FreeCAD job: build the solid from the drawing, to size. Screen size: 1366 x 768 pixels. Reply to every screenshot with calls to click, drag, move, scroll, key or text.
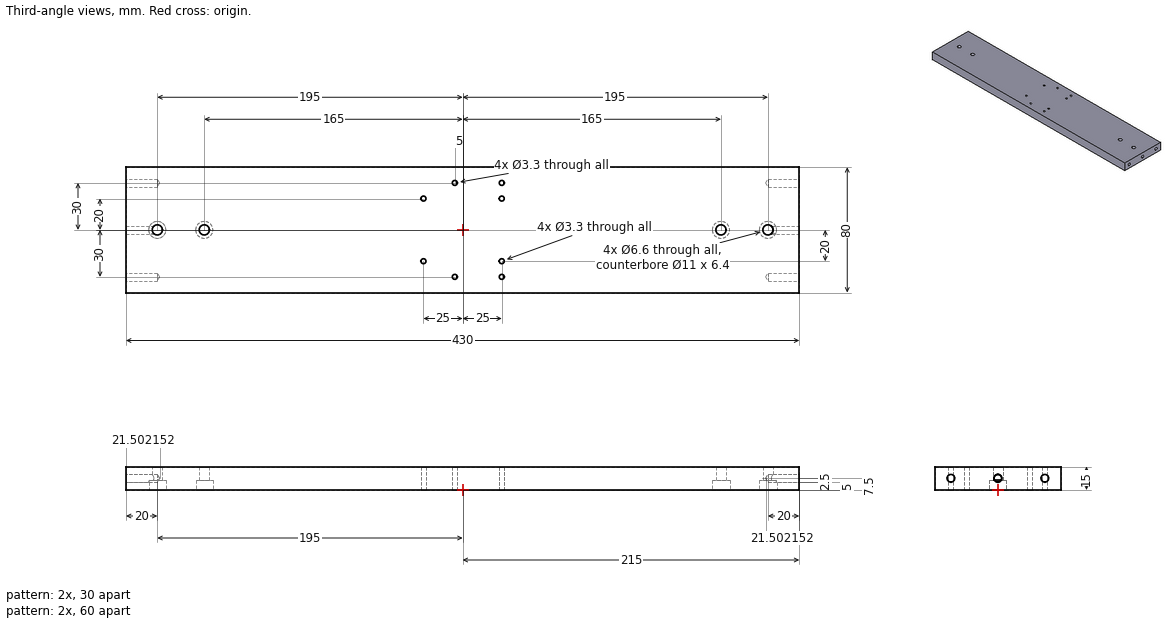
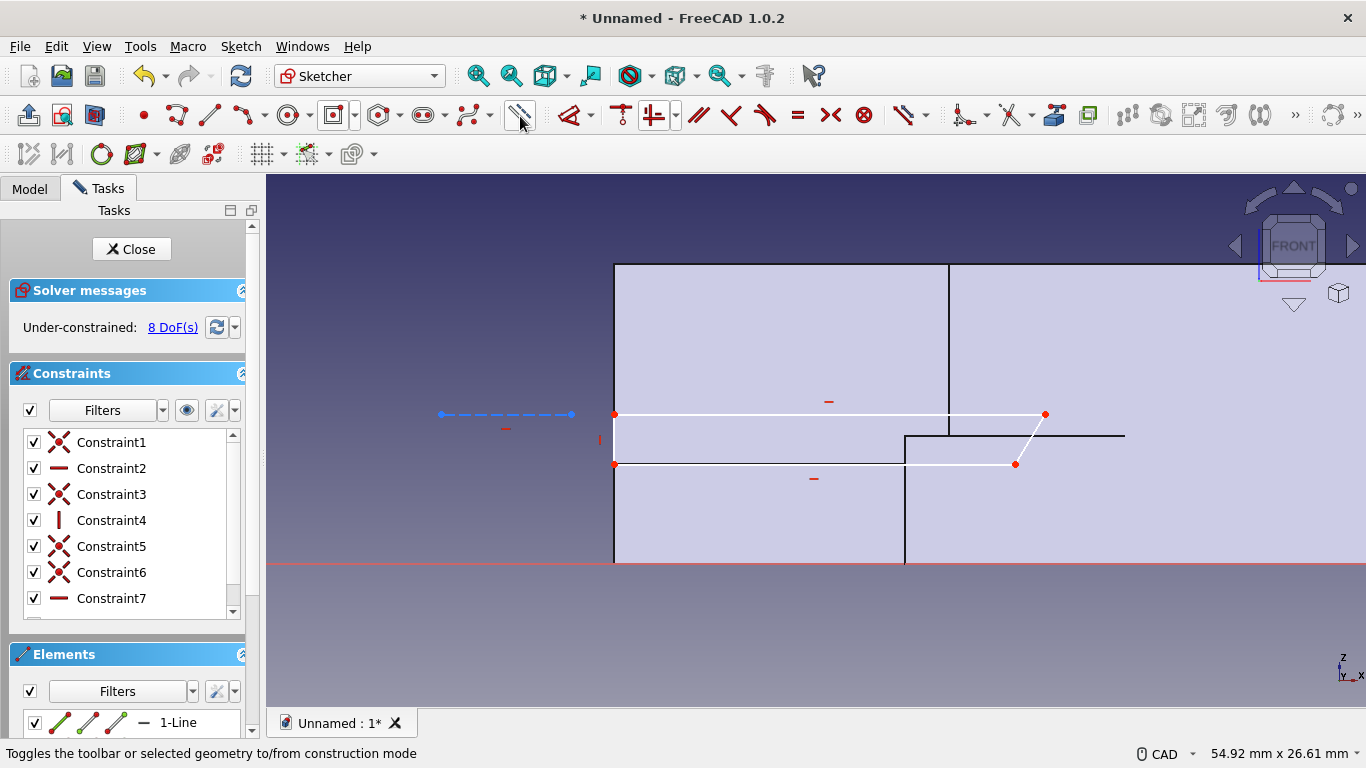
click(568, 116)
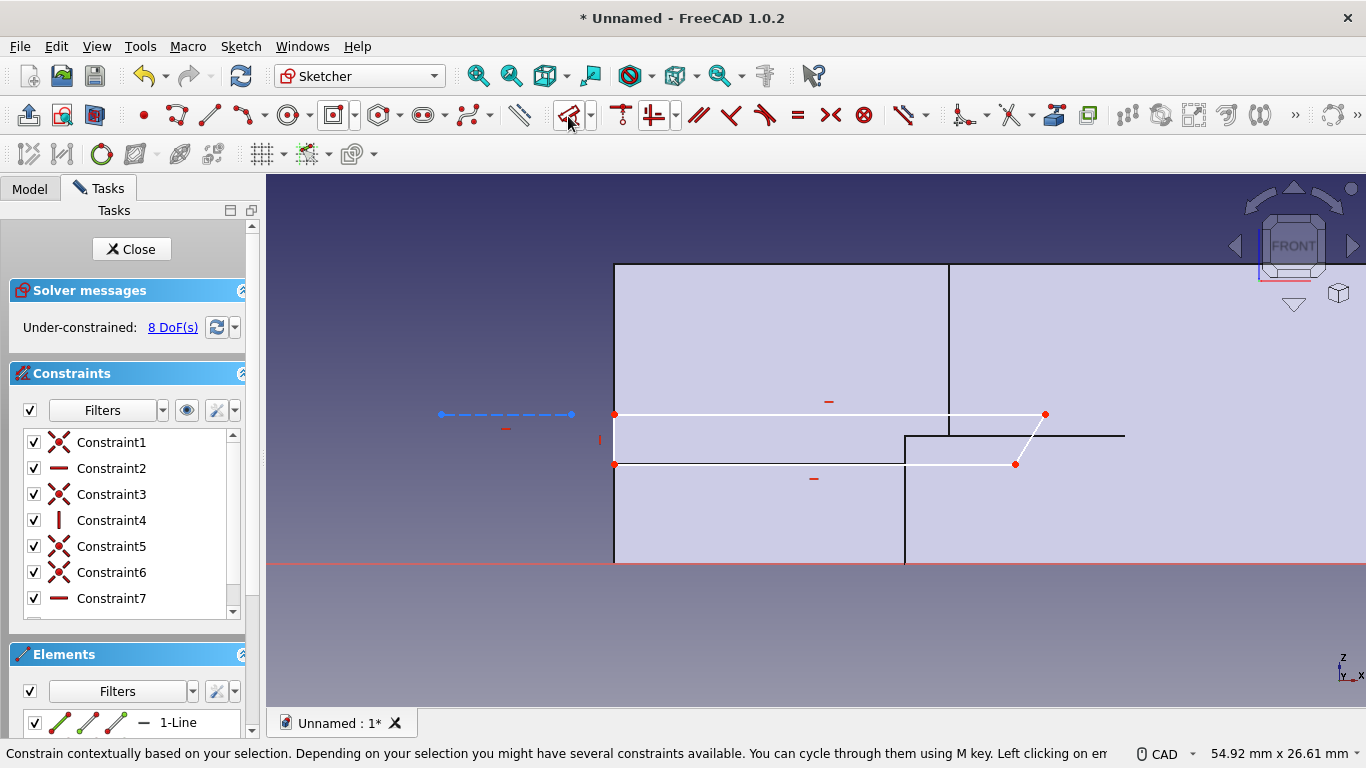
click(895, 465)
click(815, 499)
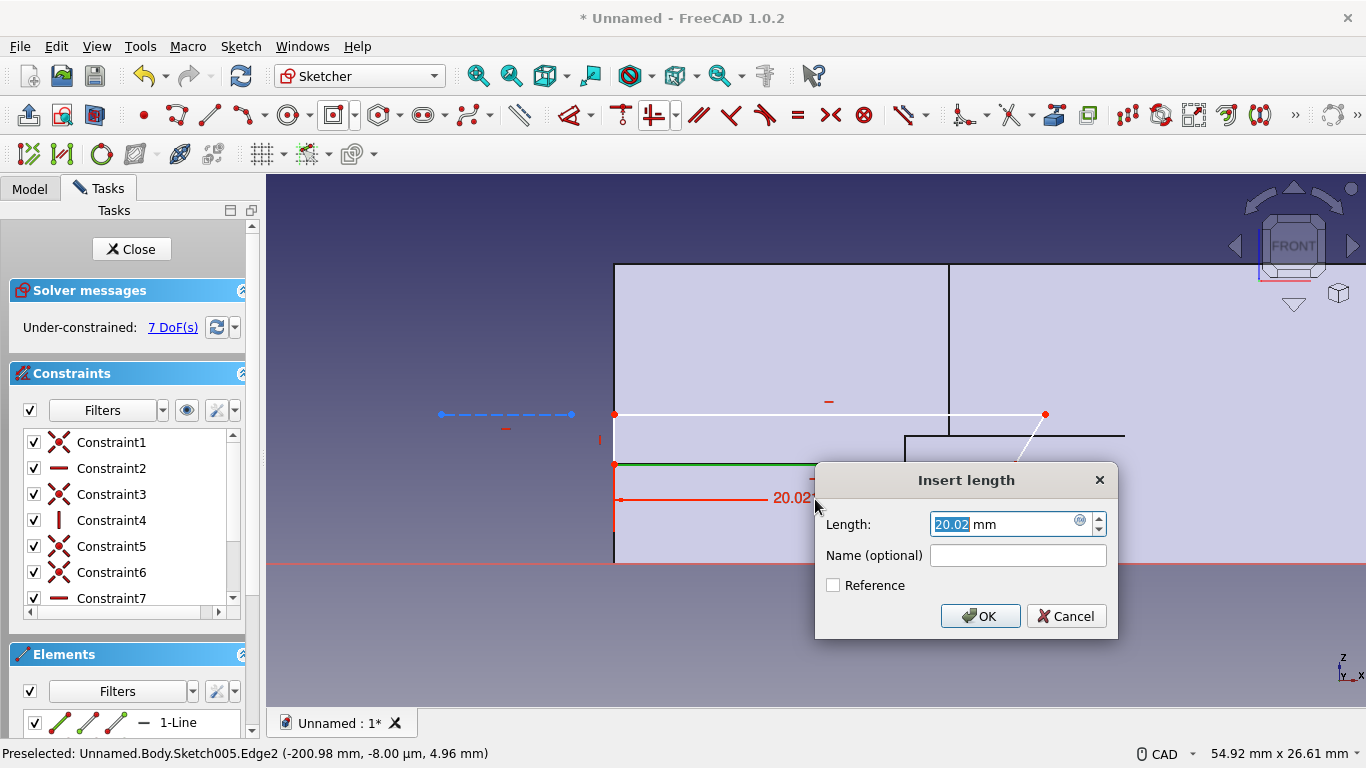
text(20)
key(Return)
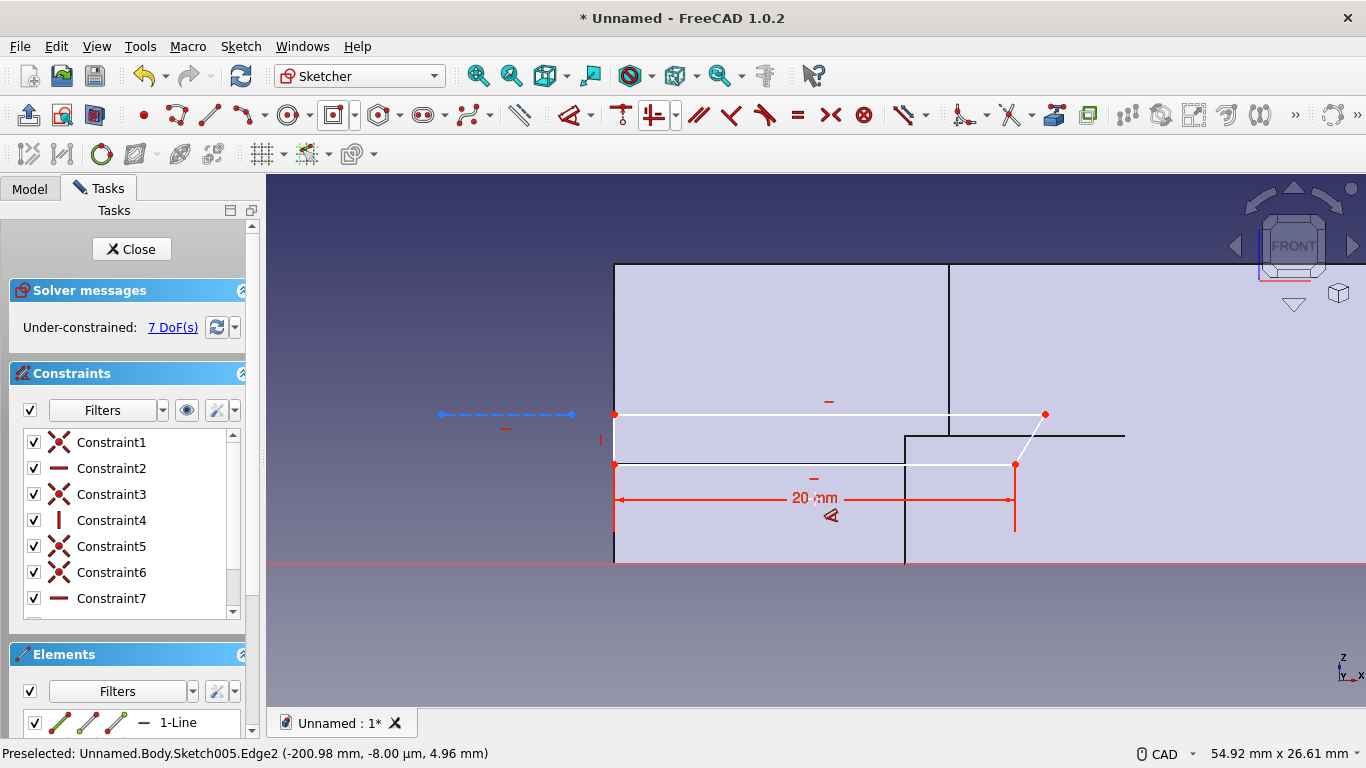
click(1015, 465)
click(981, 515)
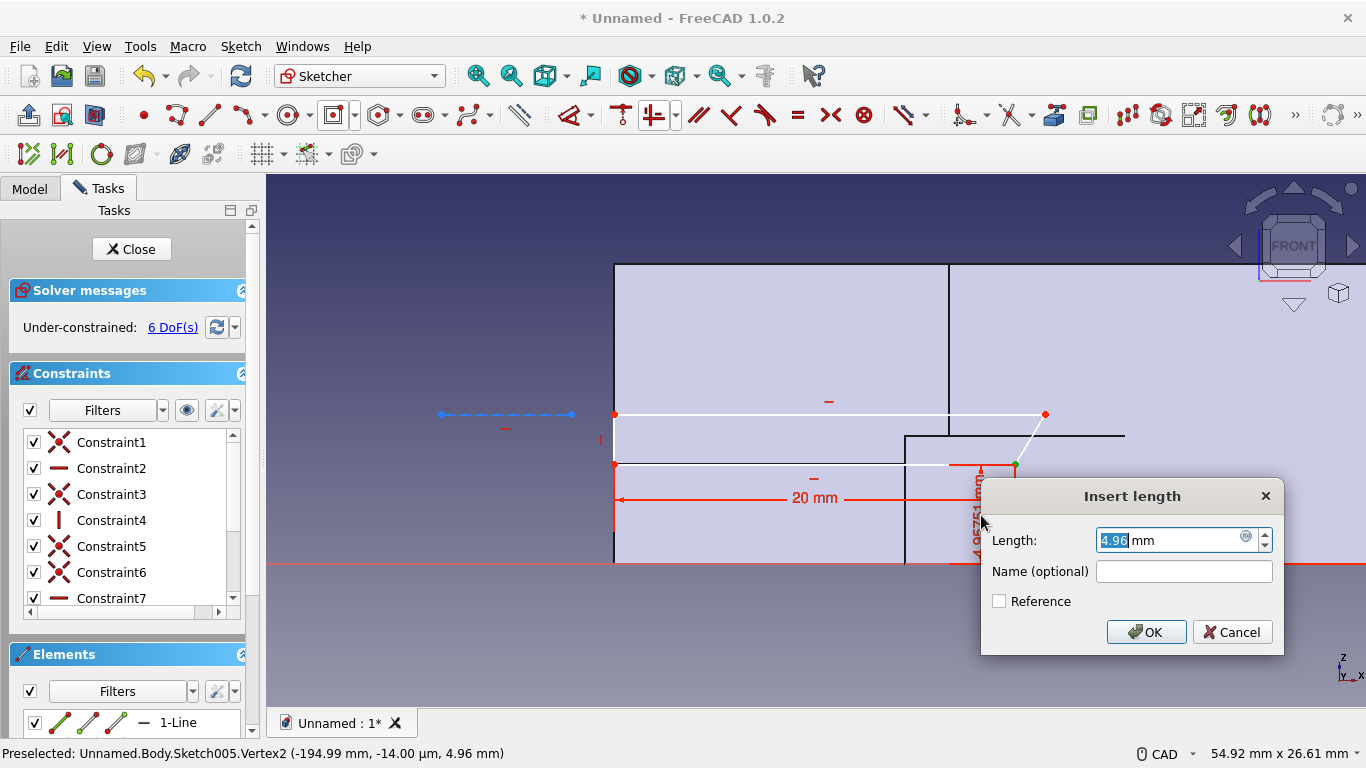
text(5)
key(Return)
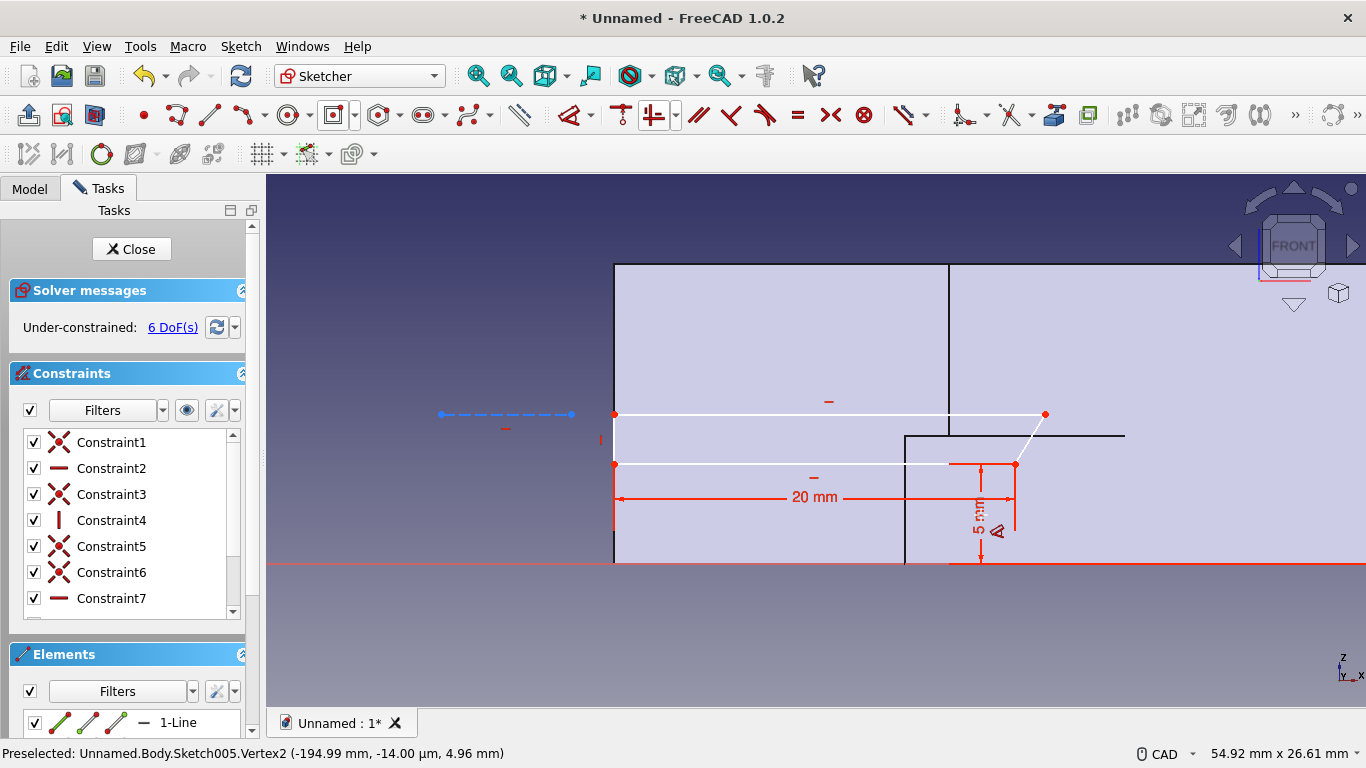
click(614, 449)
click(580, 440)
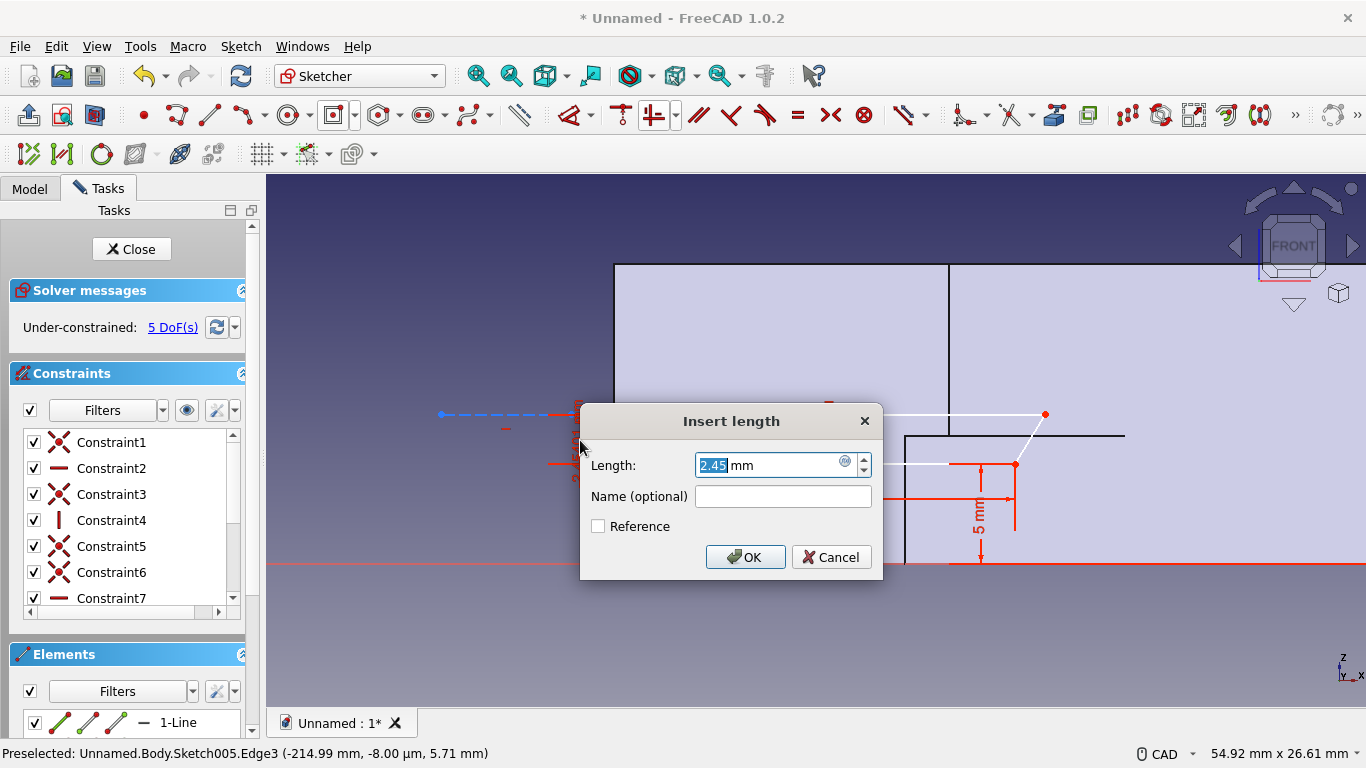
text(2.5)
key(Return)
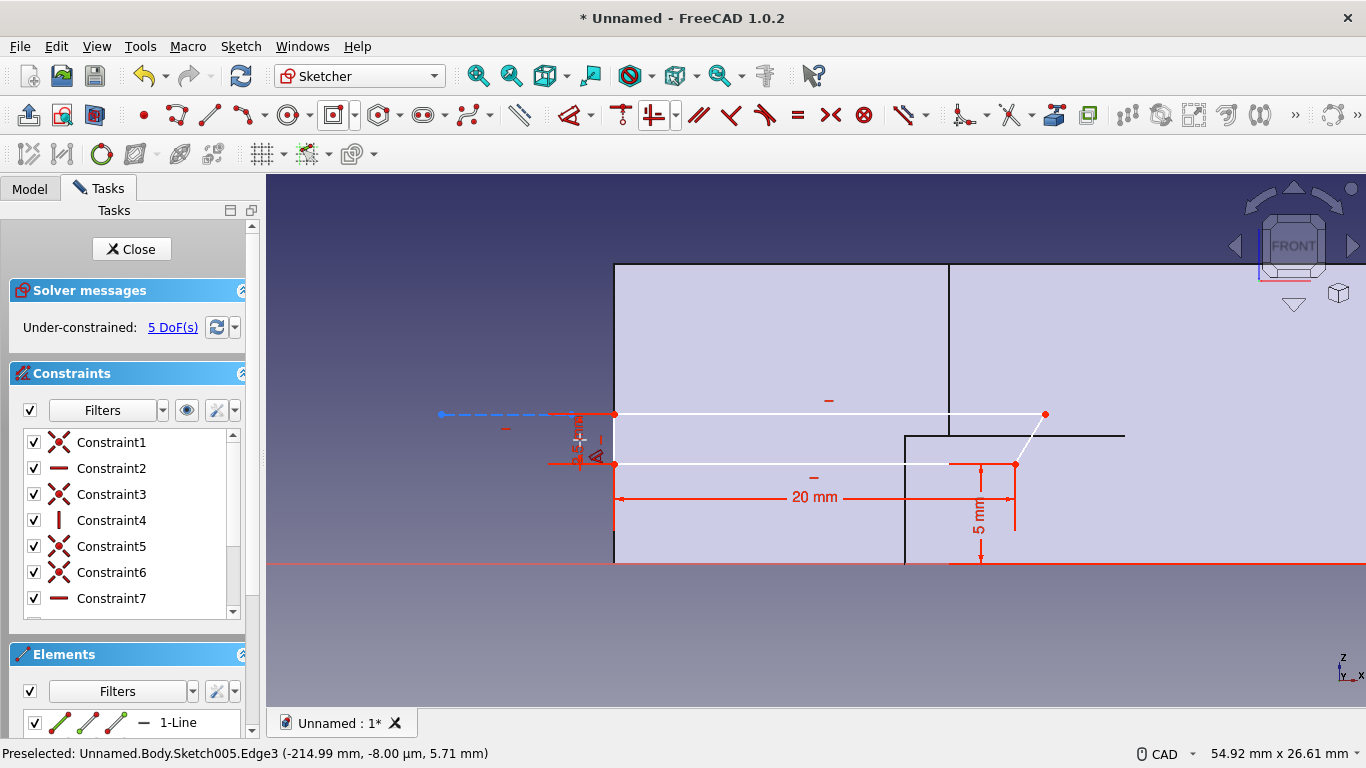
click(1015, 464)
click(1108, 598)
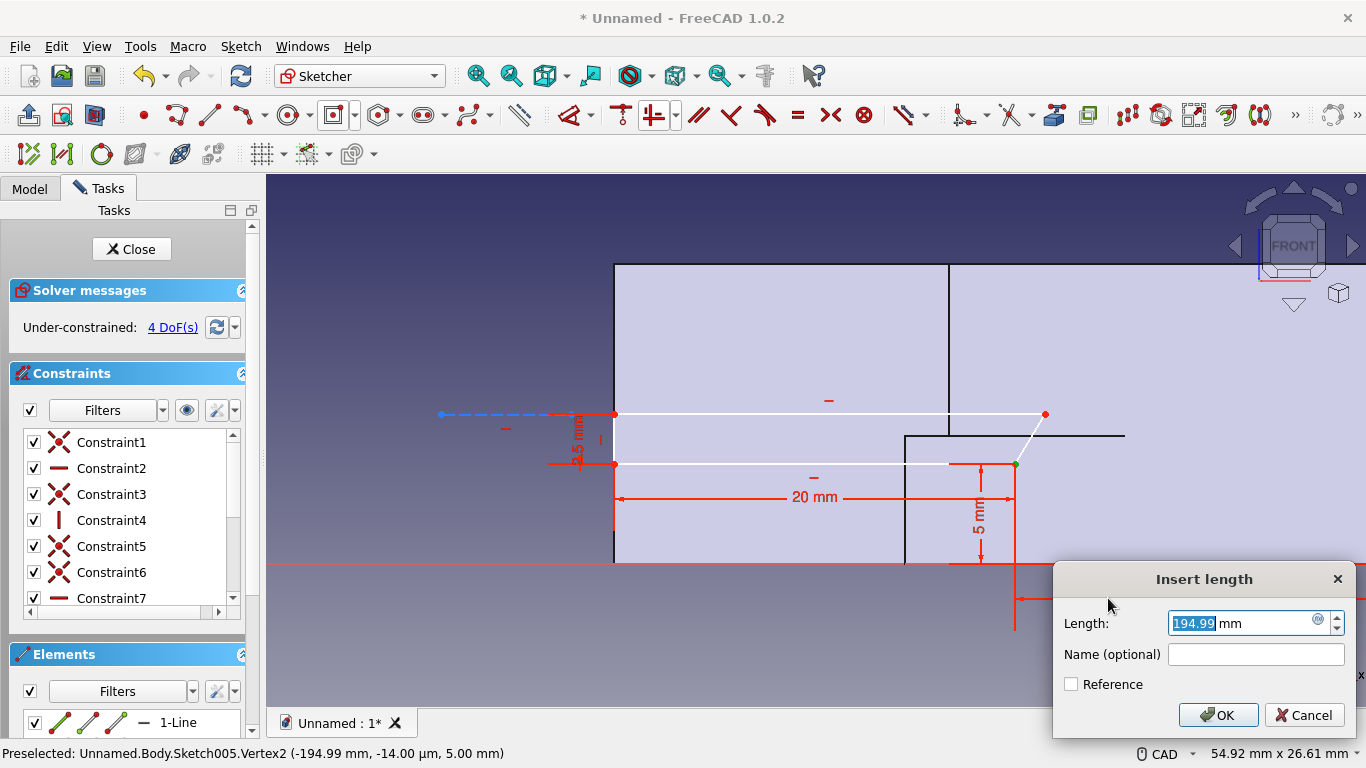
text(195)
key(Return)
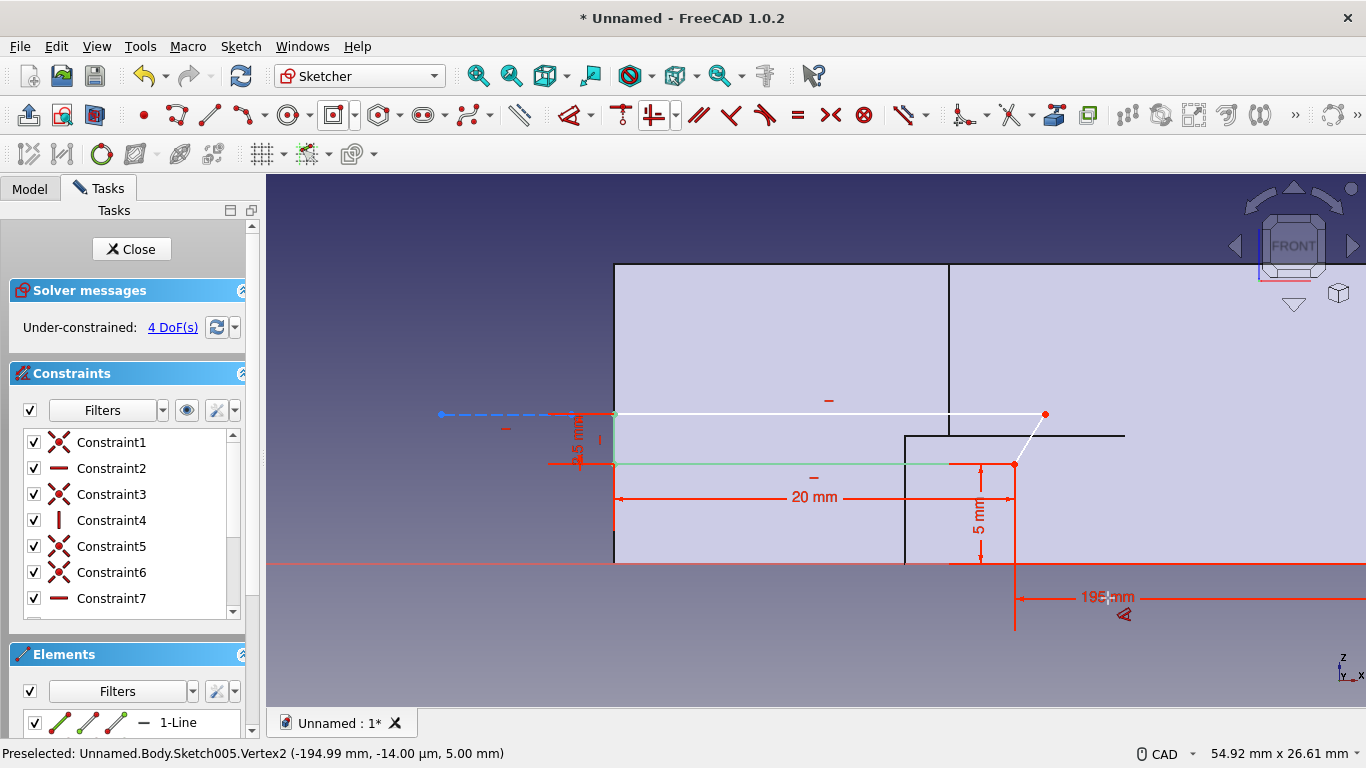
click(571, 415)
click(537, 490)